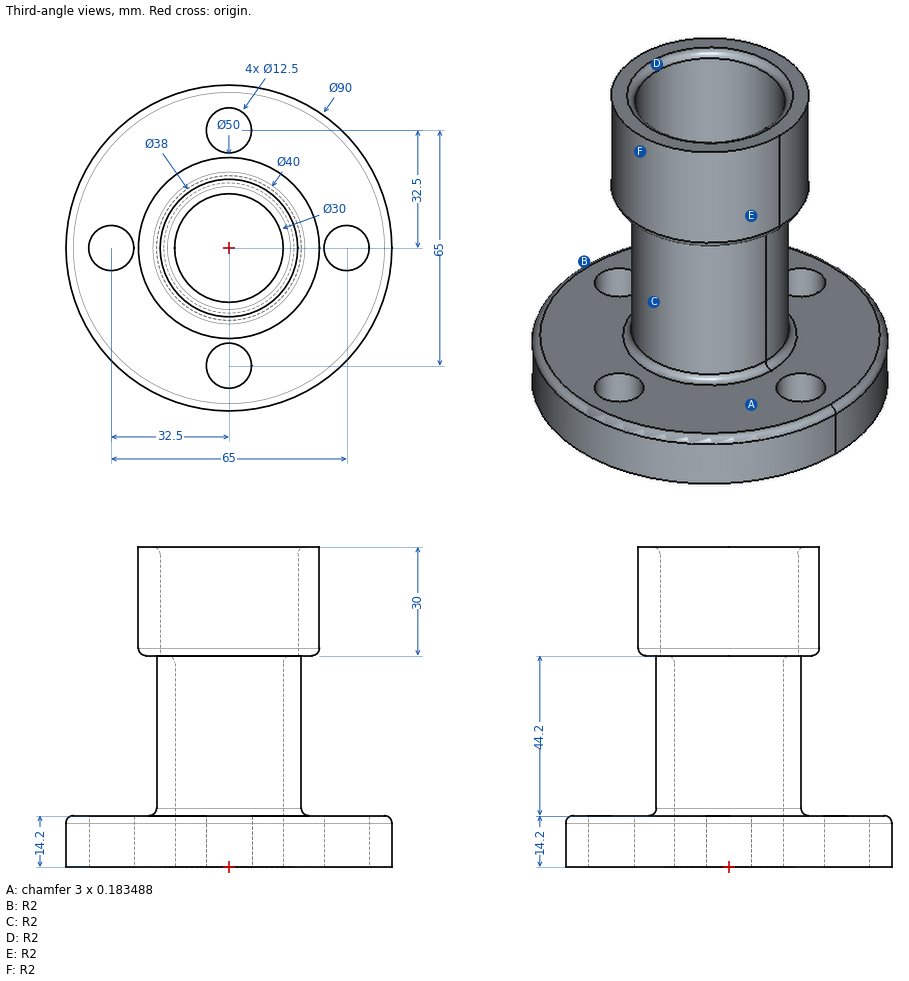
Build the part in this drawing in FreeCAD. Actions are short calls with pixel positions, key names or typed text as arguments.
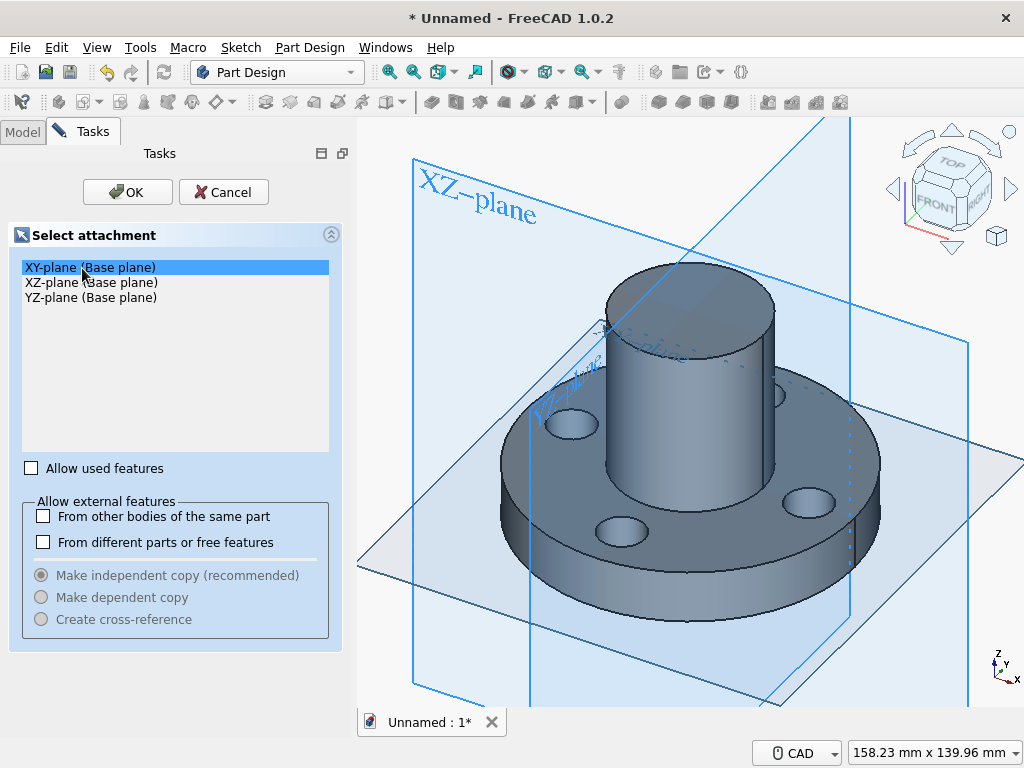
click(128, 192)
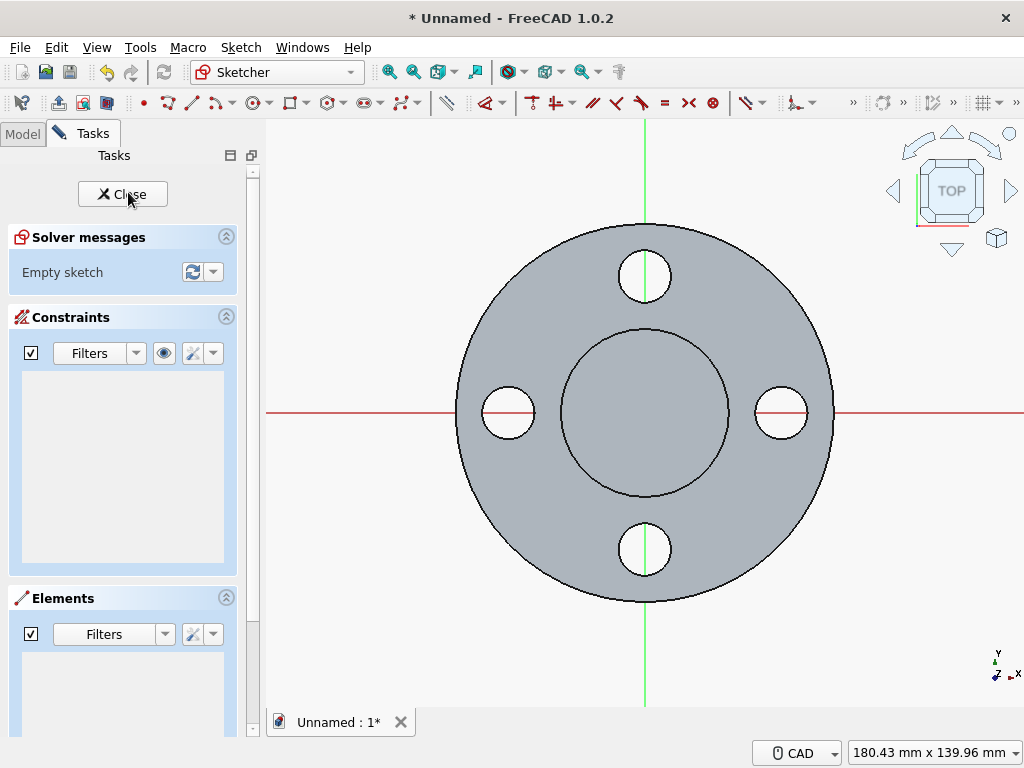
key(q)
key(s)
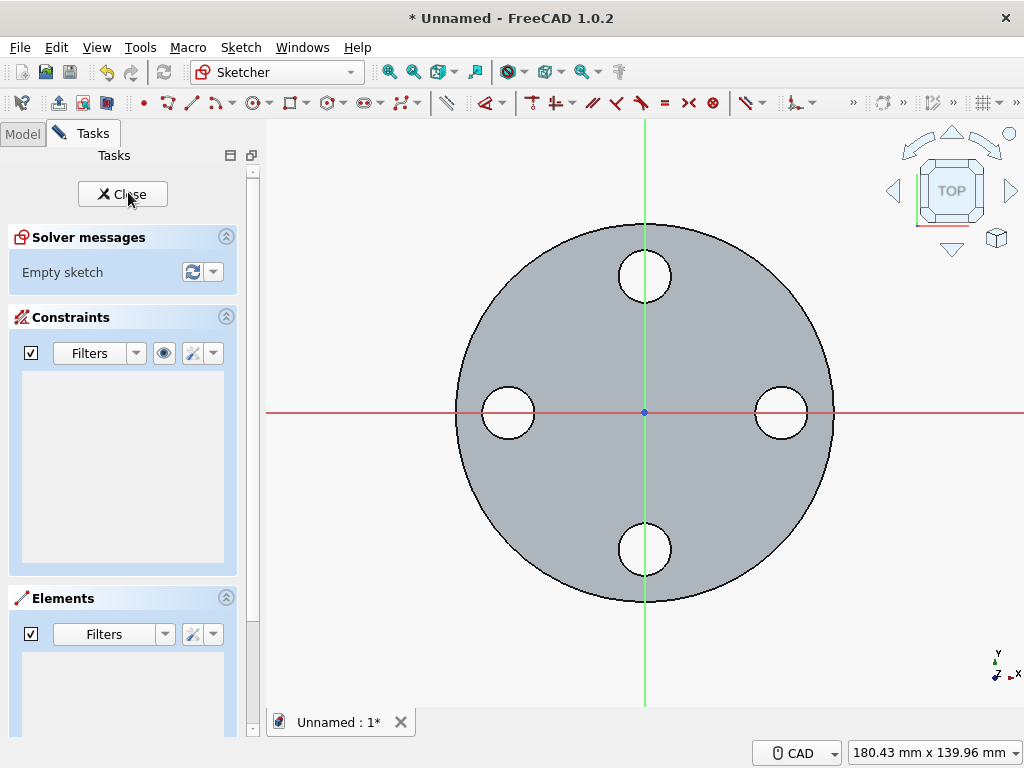
scroll(685, 413, up, 5)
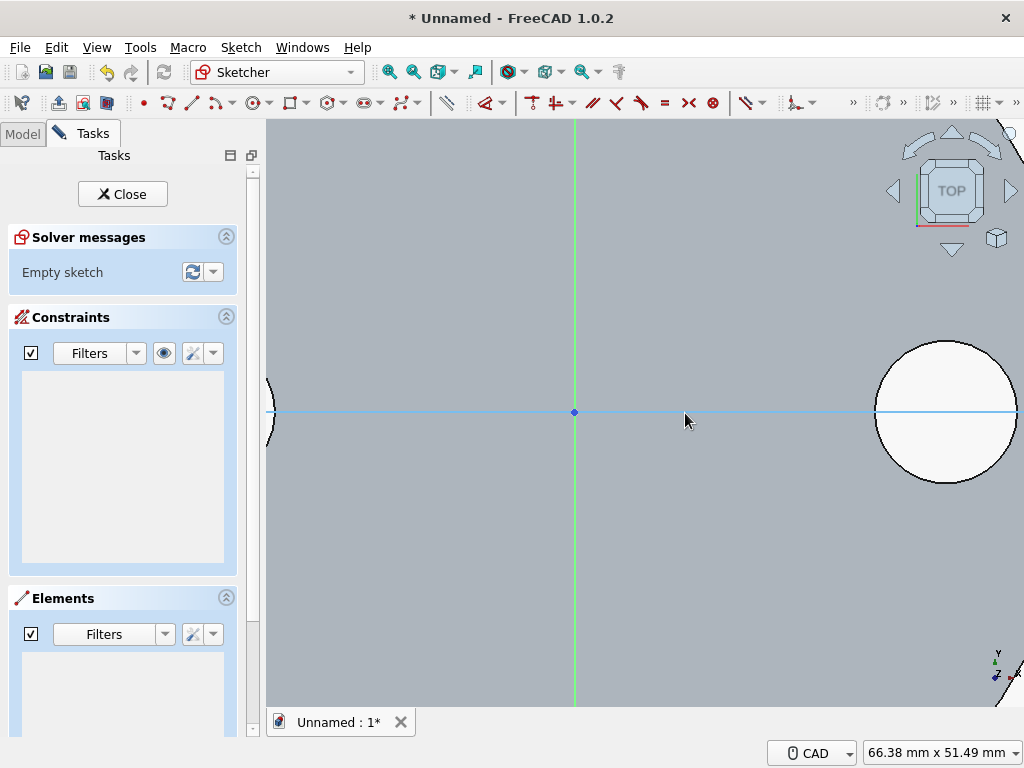
click(254, 104)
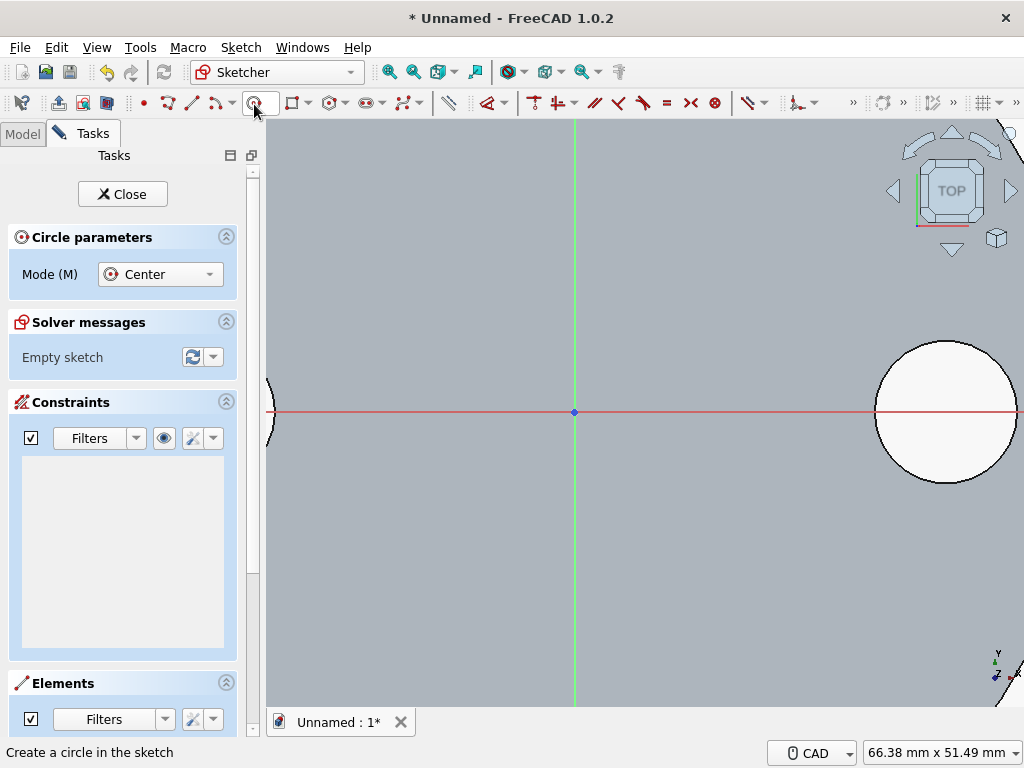
click(575, 412)
move(696, 291)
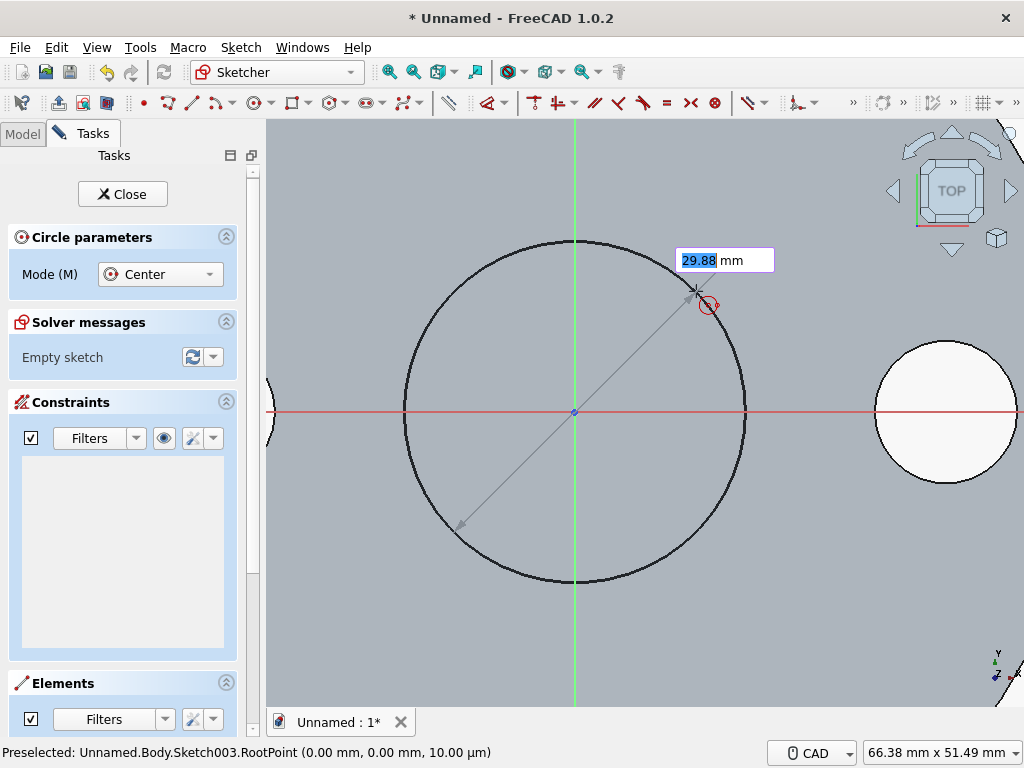
text(30)
key(Return)
key(Escape)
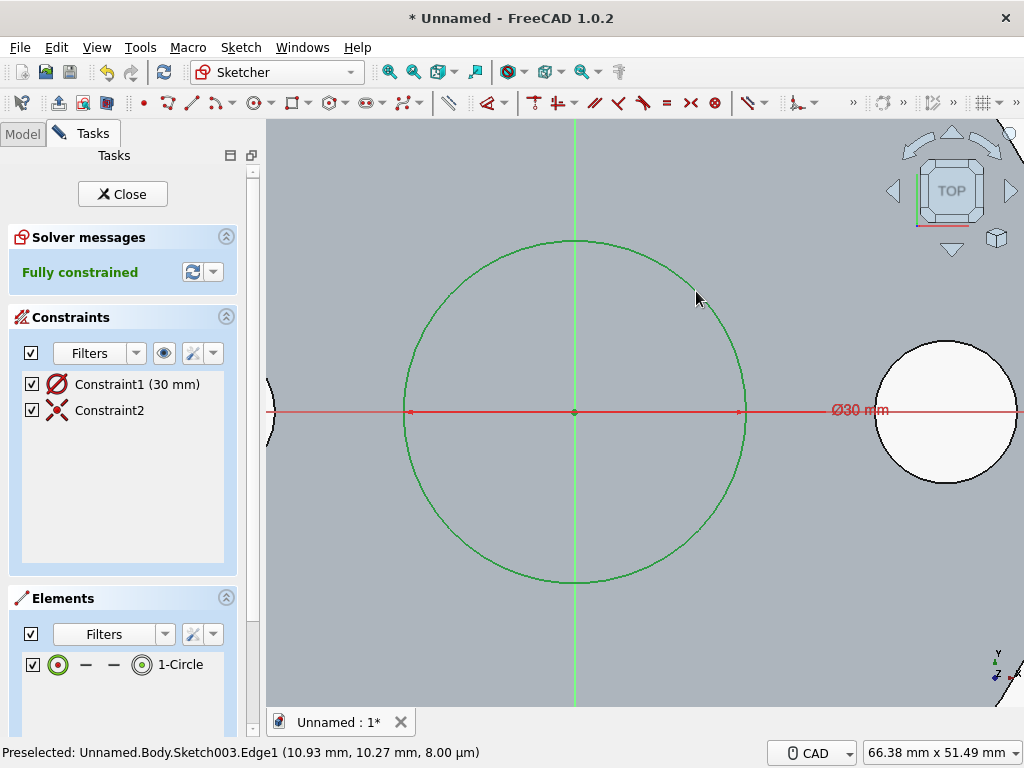
click(123, 194)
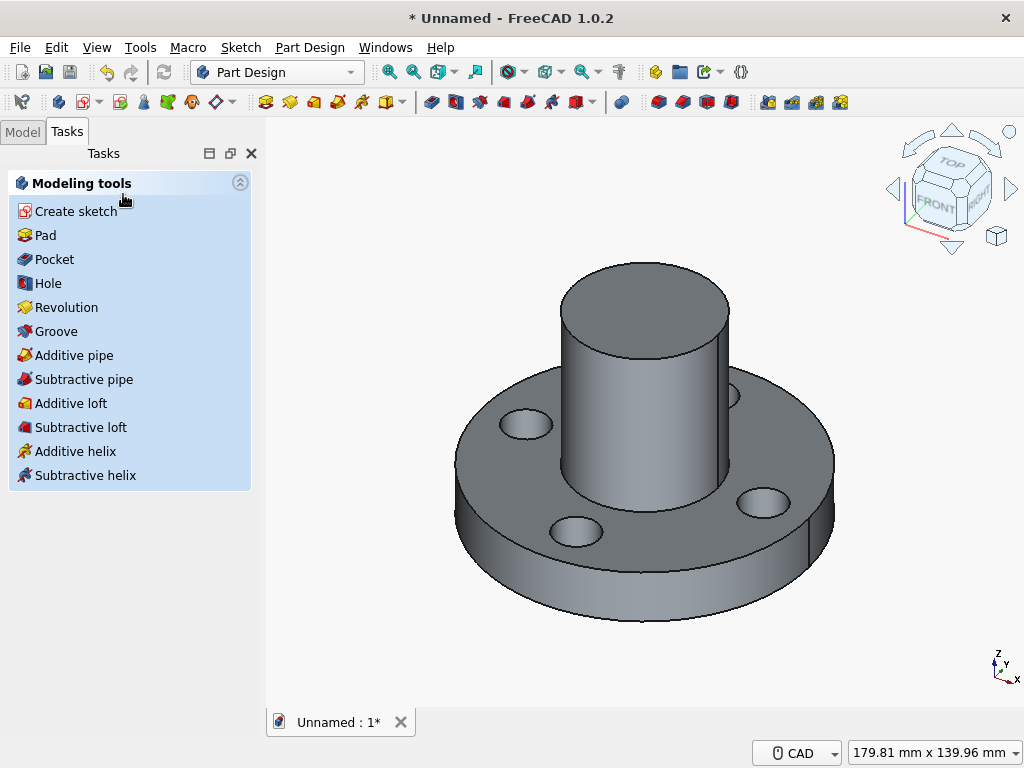
click(432, 102)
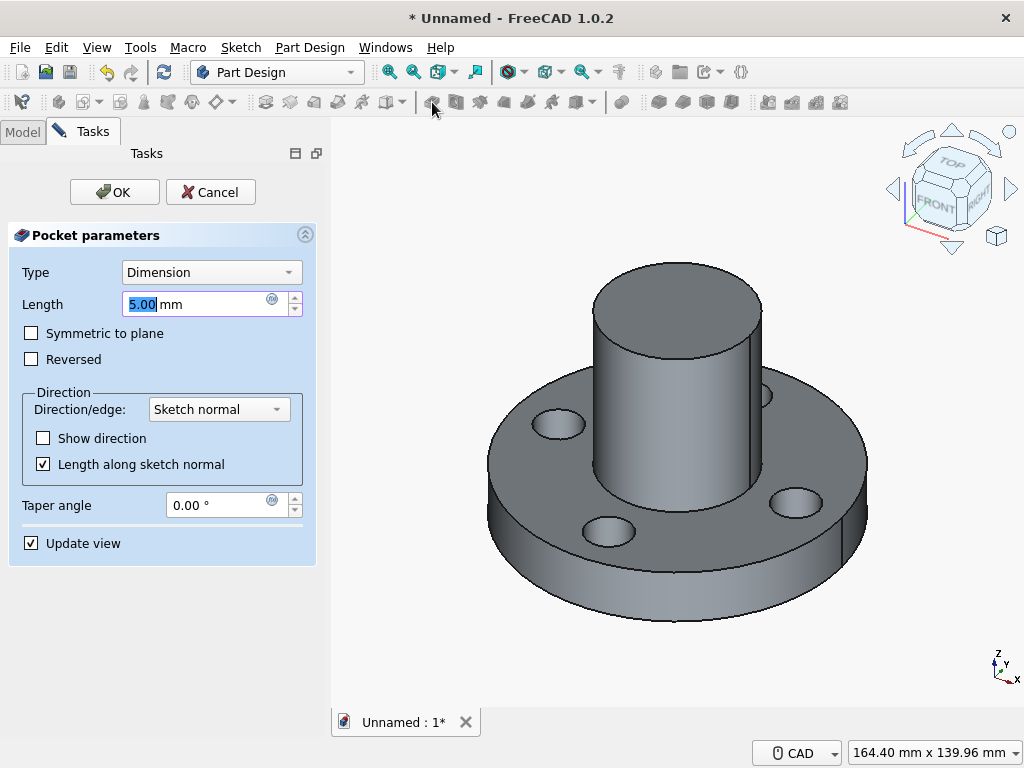
click(212, 272)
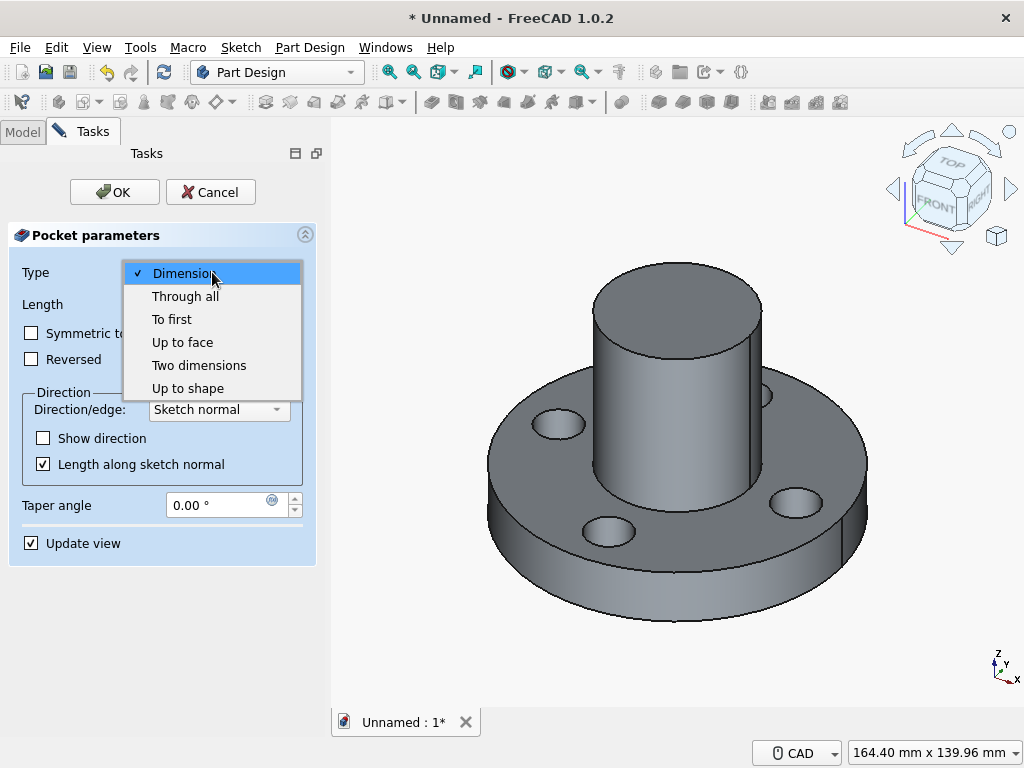
click(212, 296)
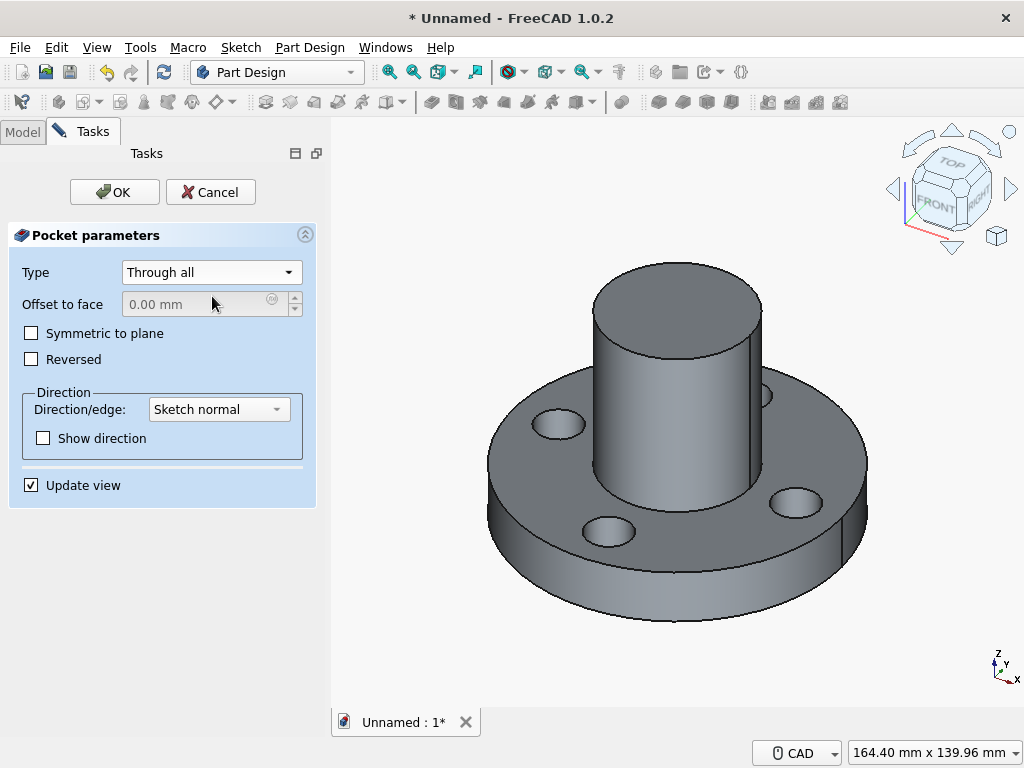
click(30, 359)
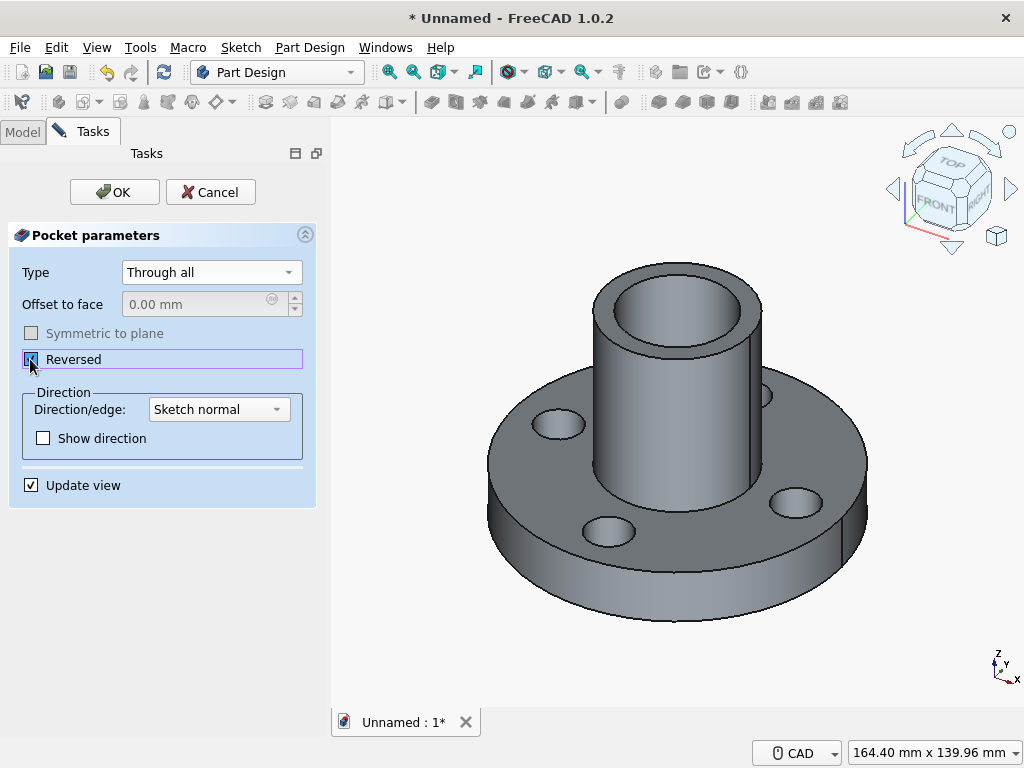
click(115, 192)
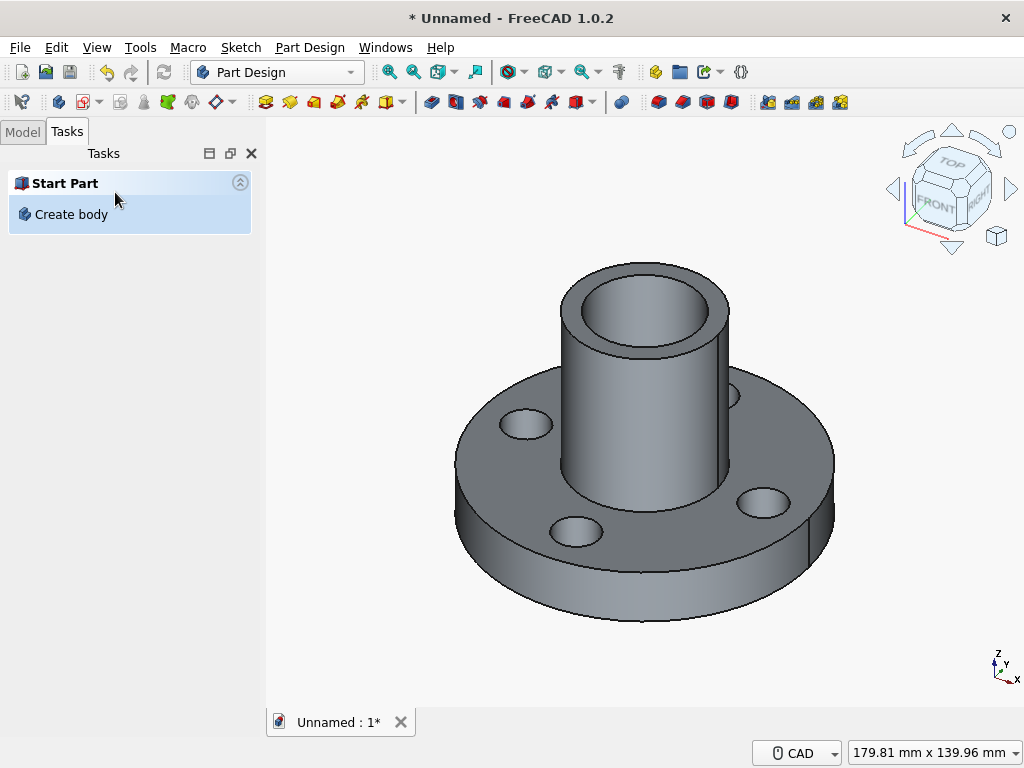
key(0)